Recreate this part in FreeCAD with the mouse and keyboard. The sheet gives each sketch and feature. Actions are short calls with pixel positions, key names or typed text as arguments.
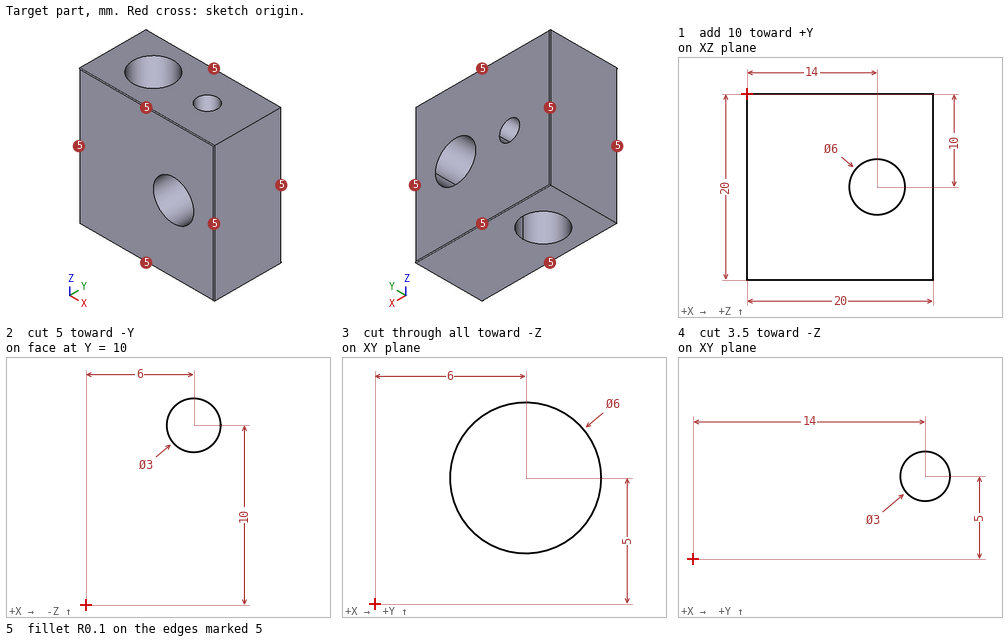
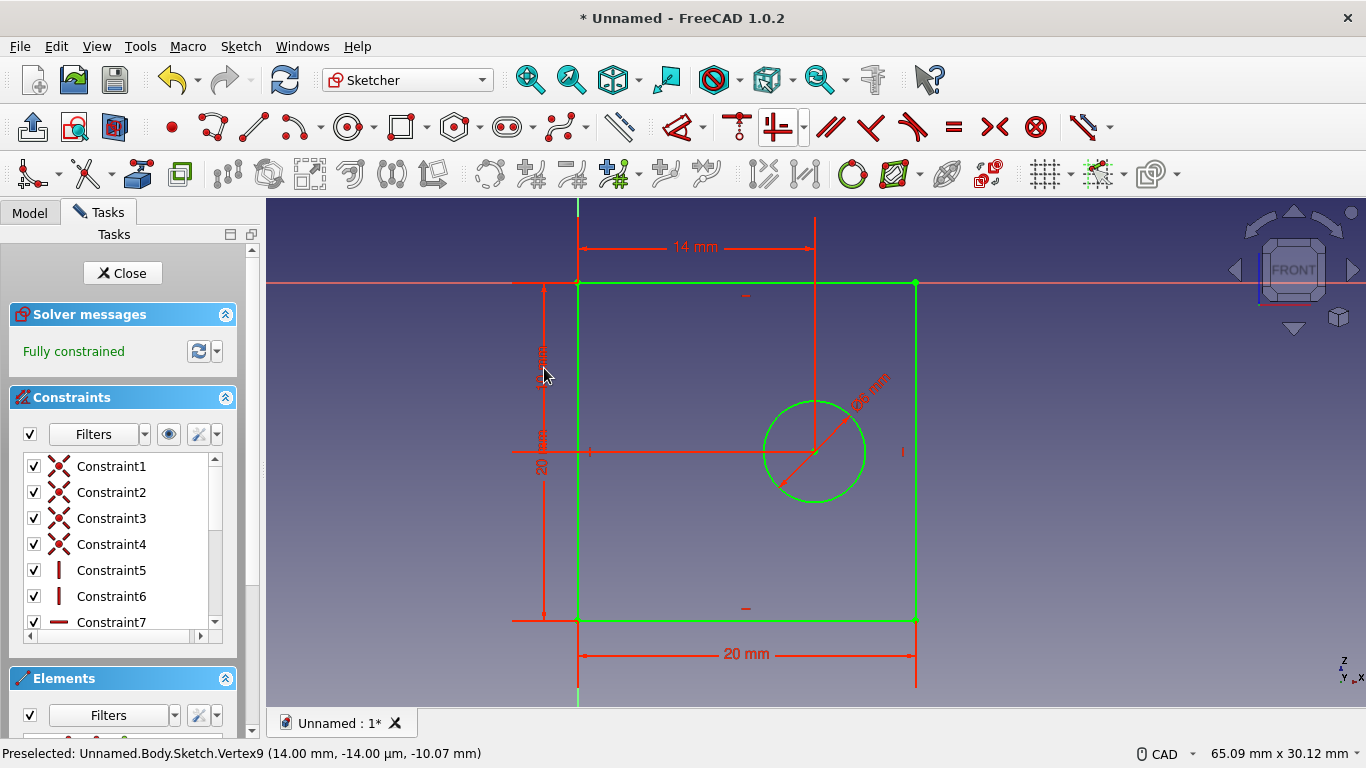
click(123, 273)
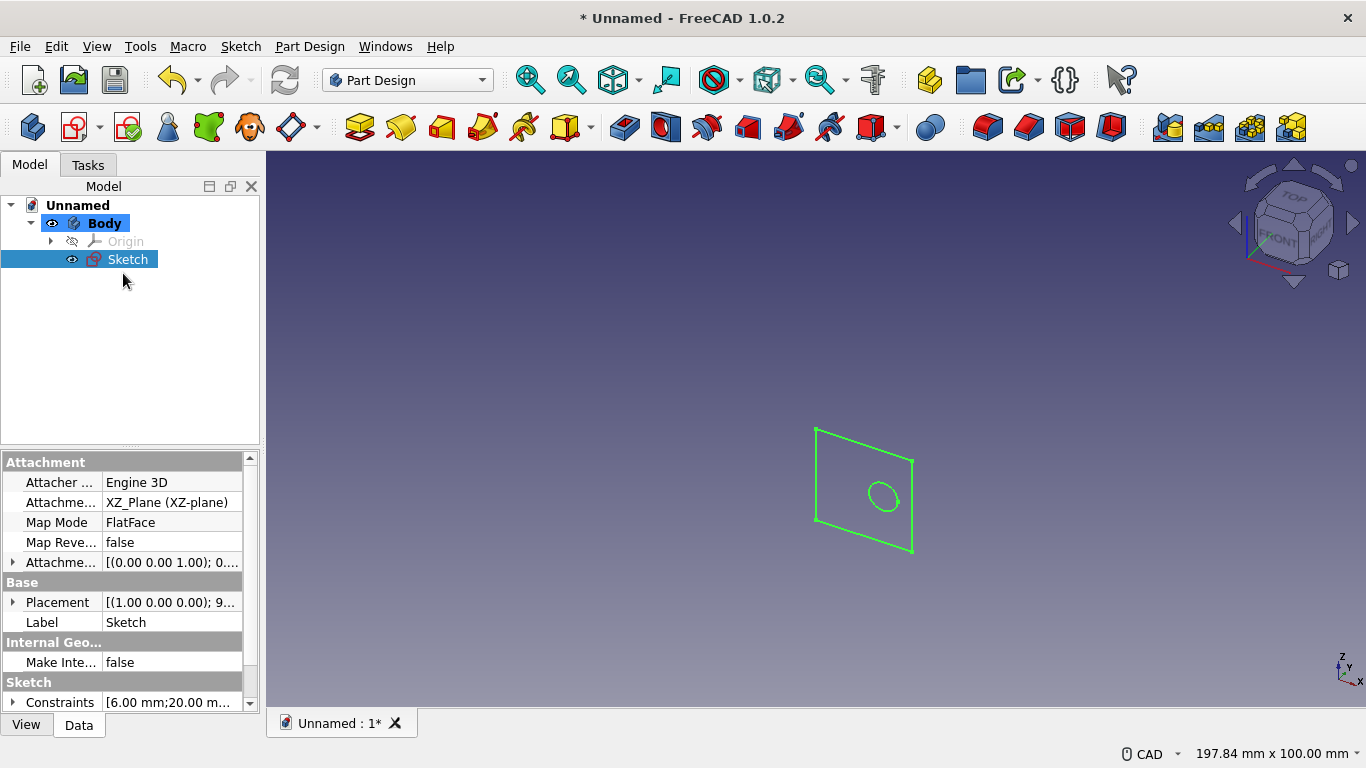
click(360, 128)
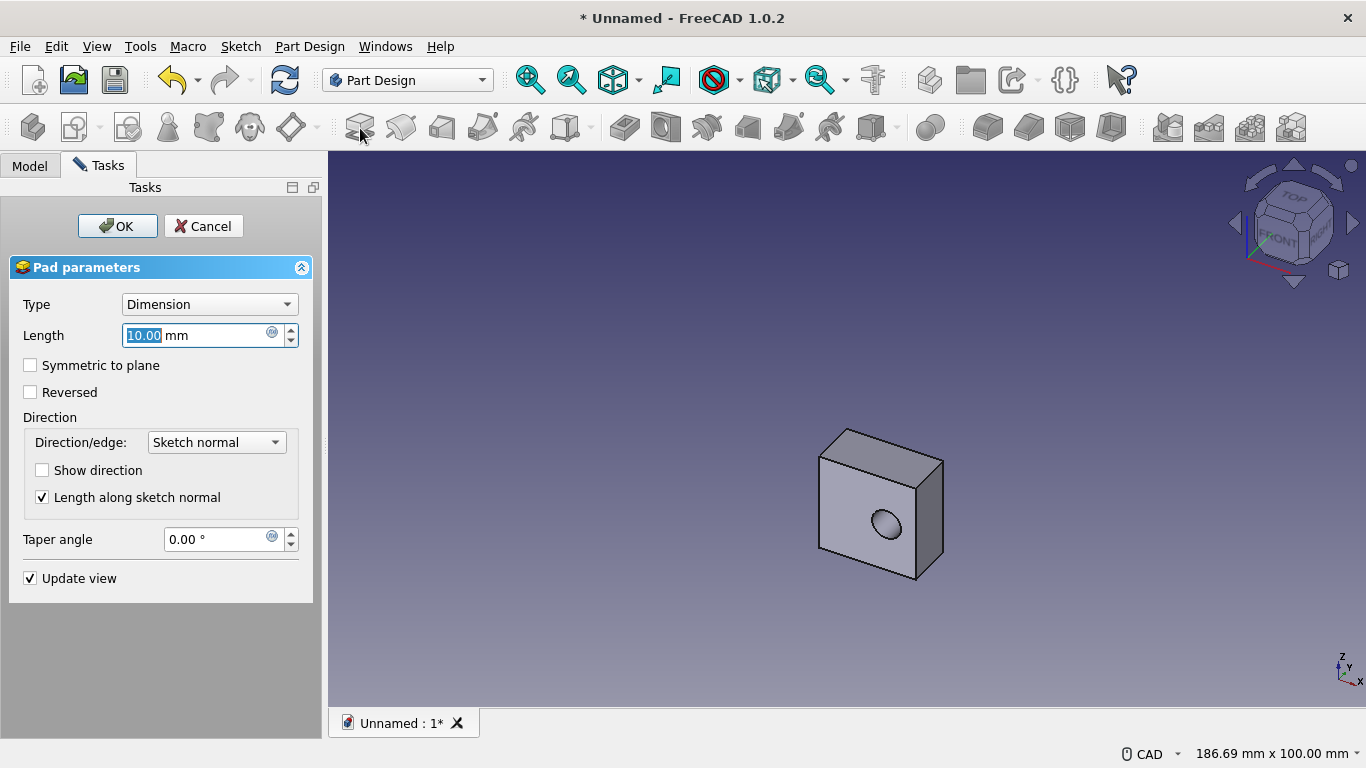
text(10)
key(Tab)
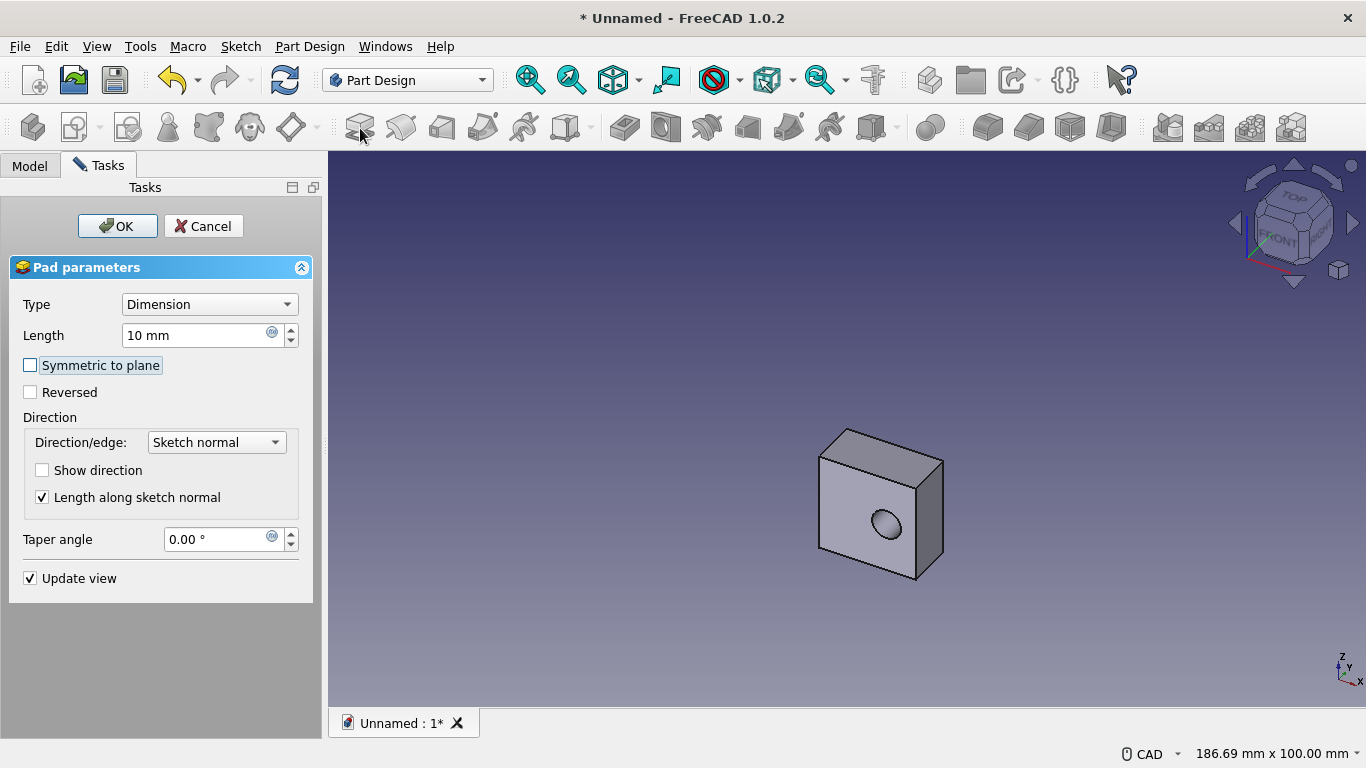
click(31, 392)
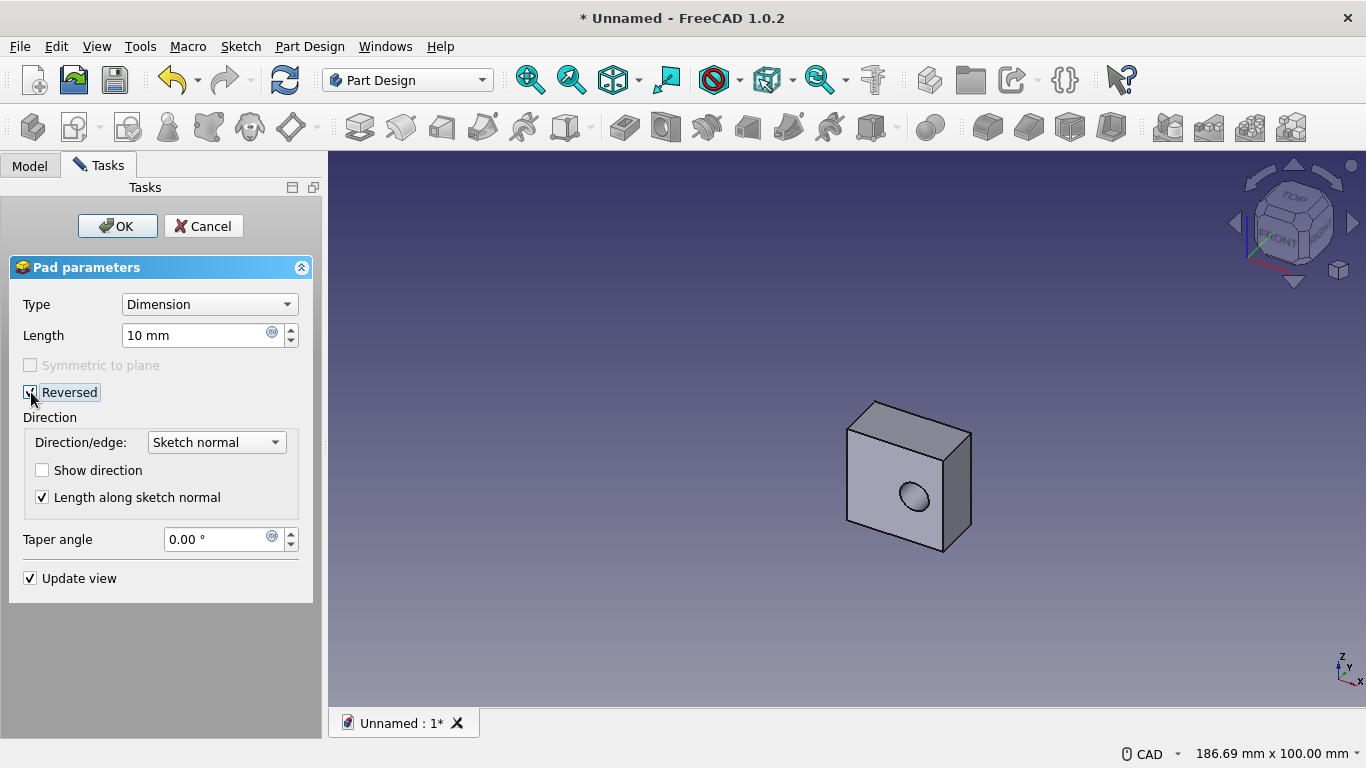
click(118, 226)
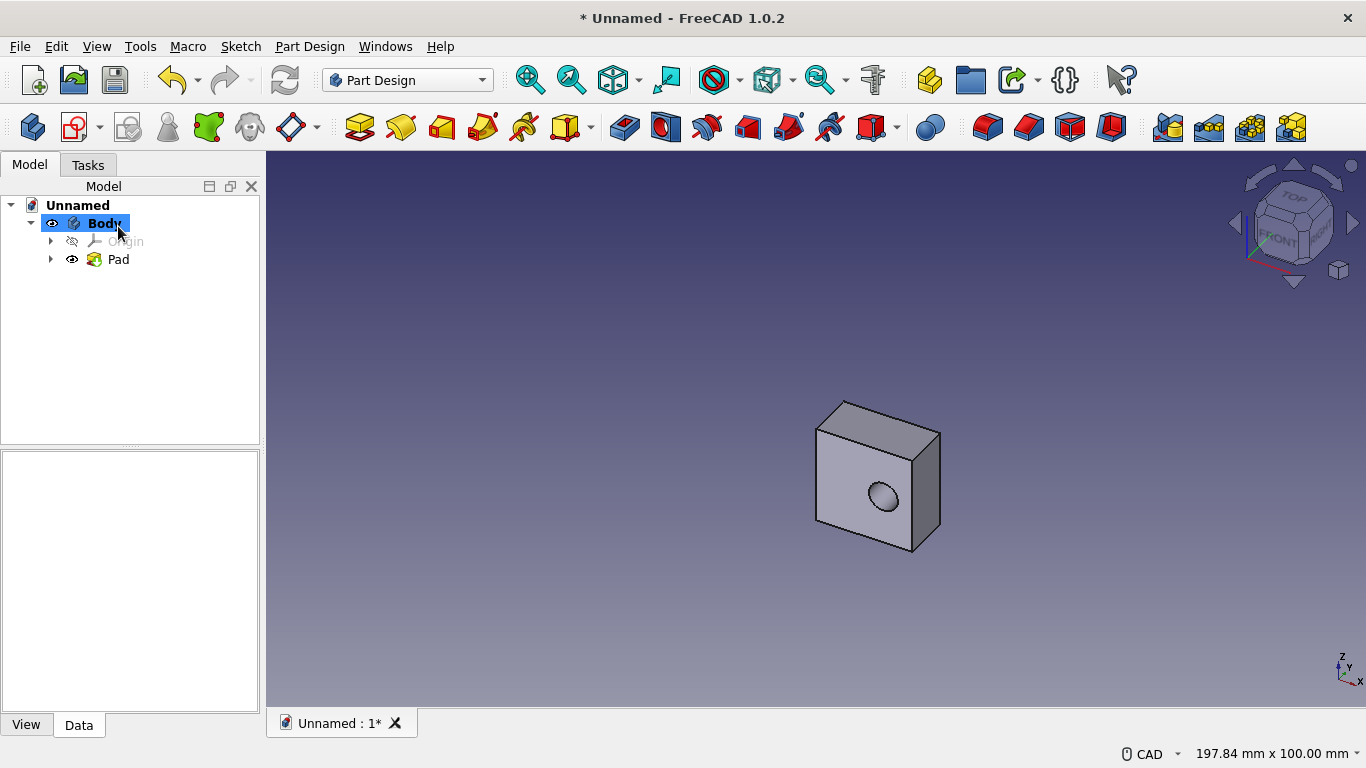
click(531, 80)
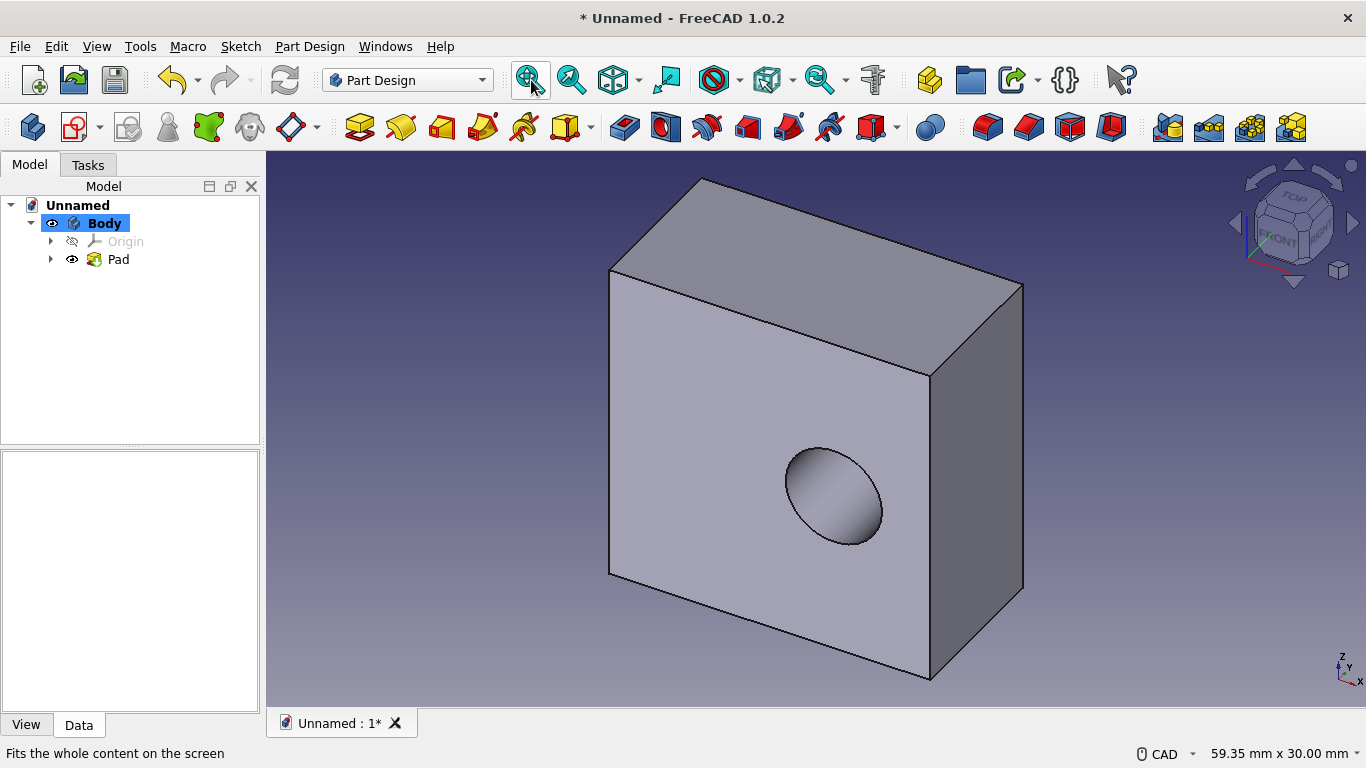
key(4)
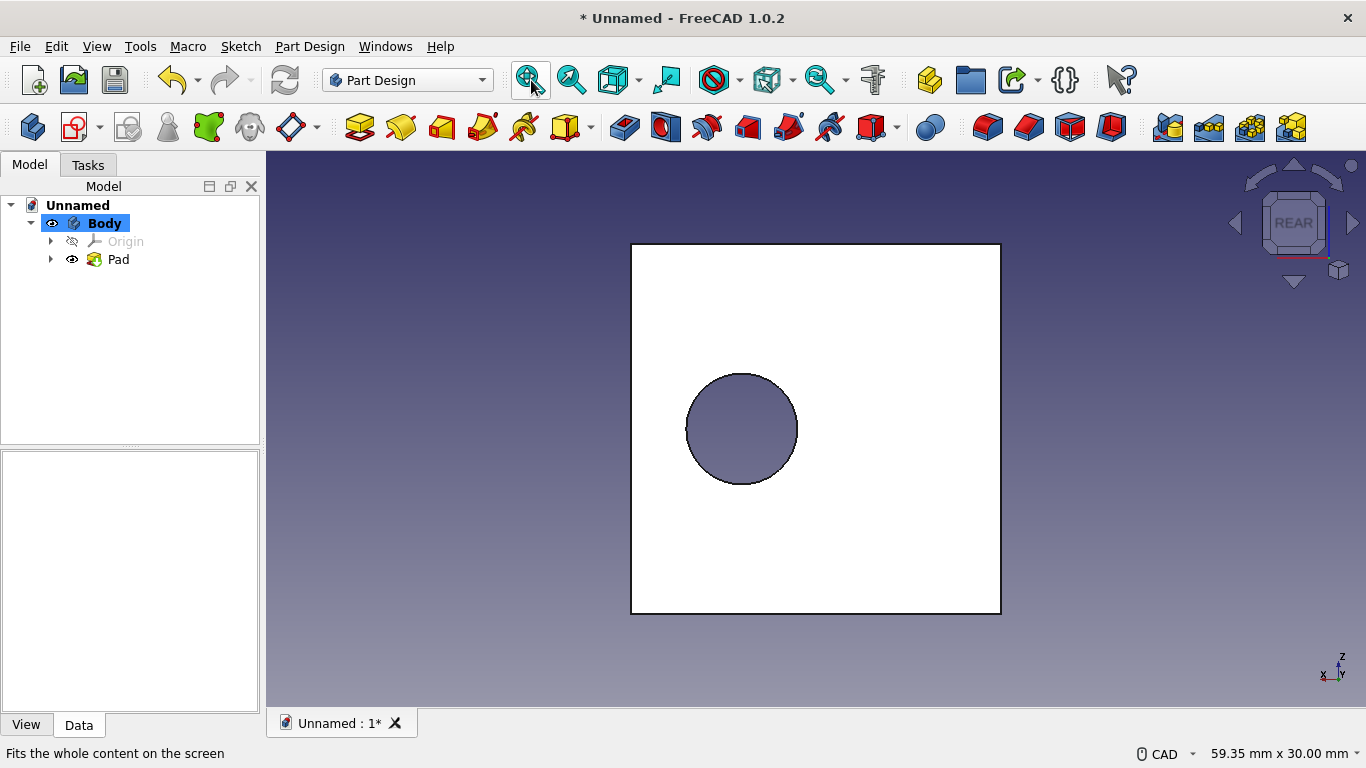
click(869, 375)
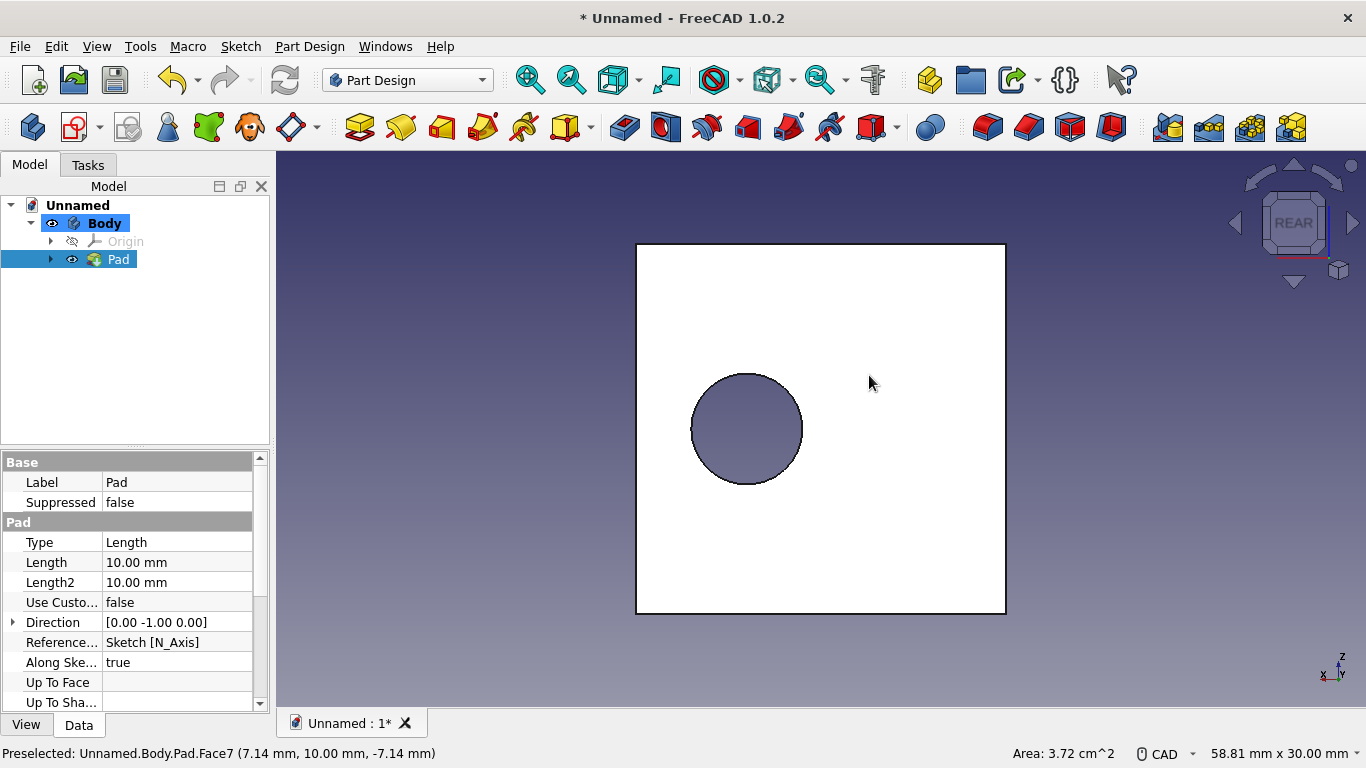
click(74, 128)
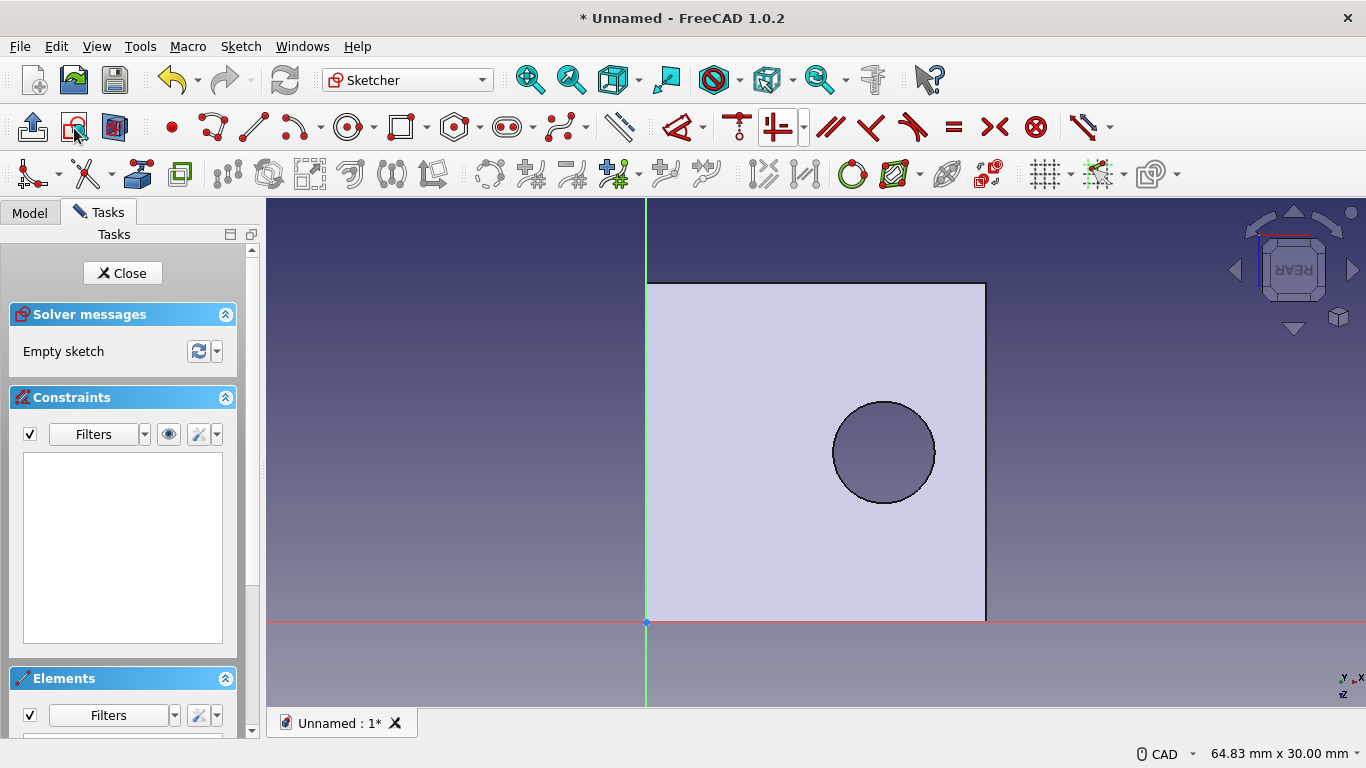
scroll(748, 452, up, 9)